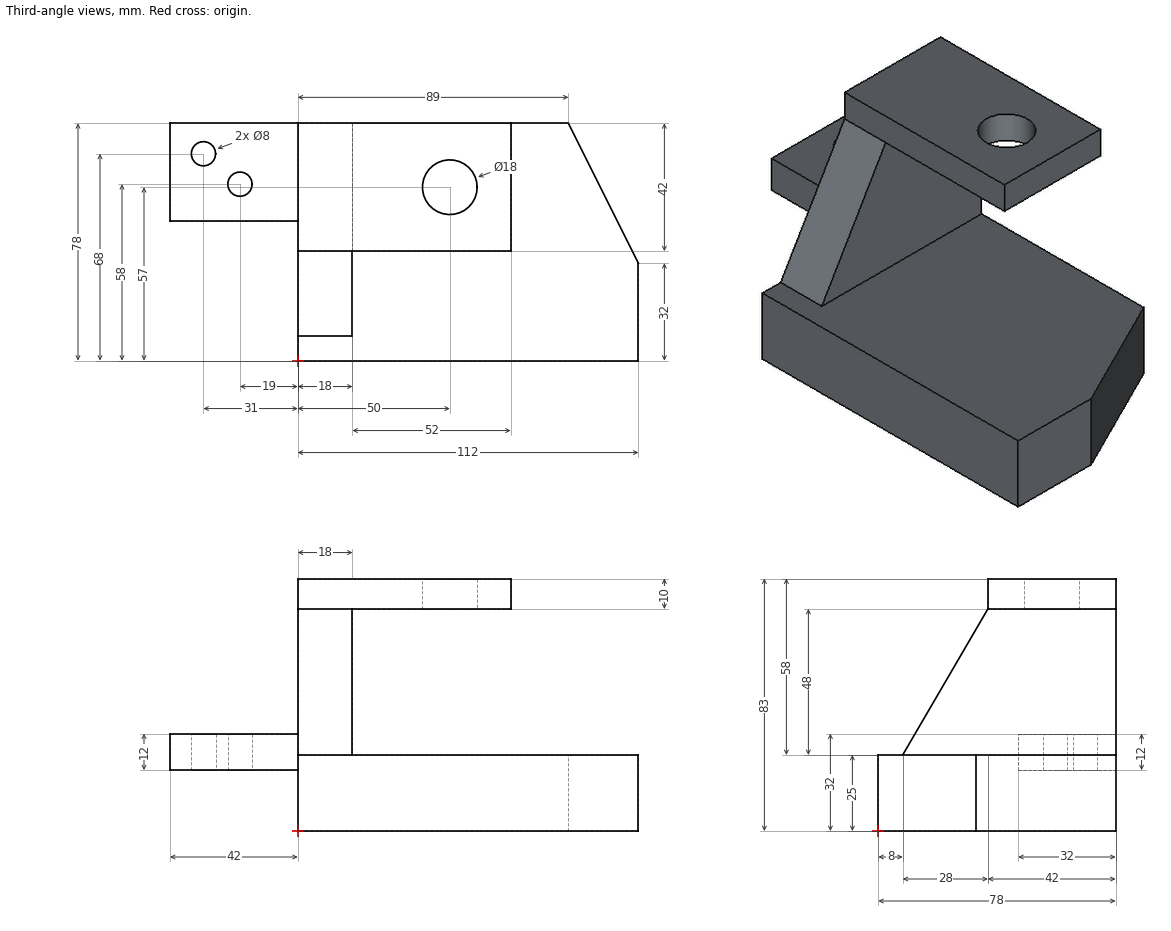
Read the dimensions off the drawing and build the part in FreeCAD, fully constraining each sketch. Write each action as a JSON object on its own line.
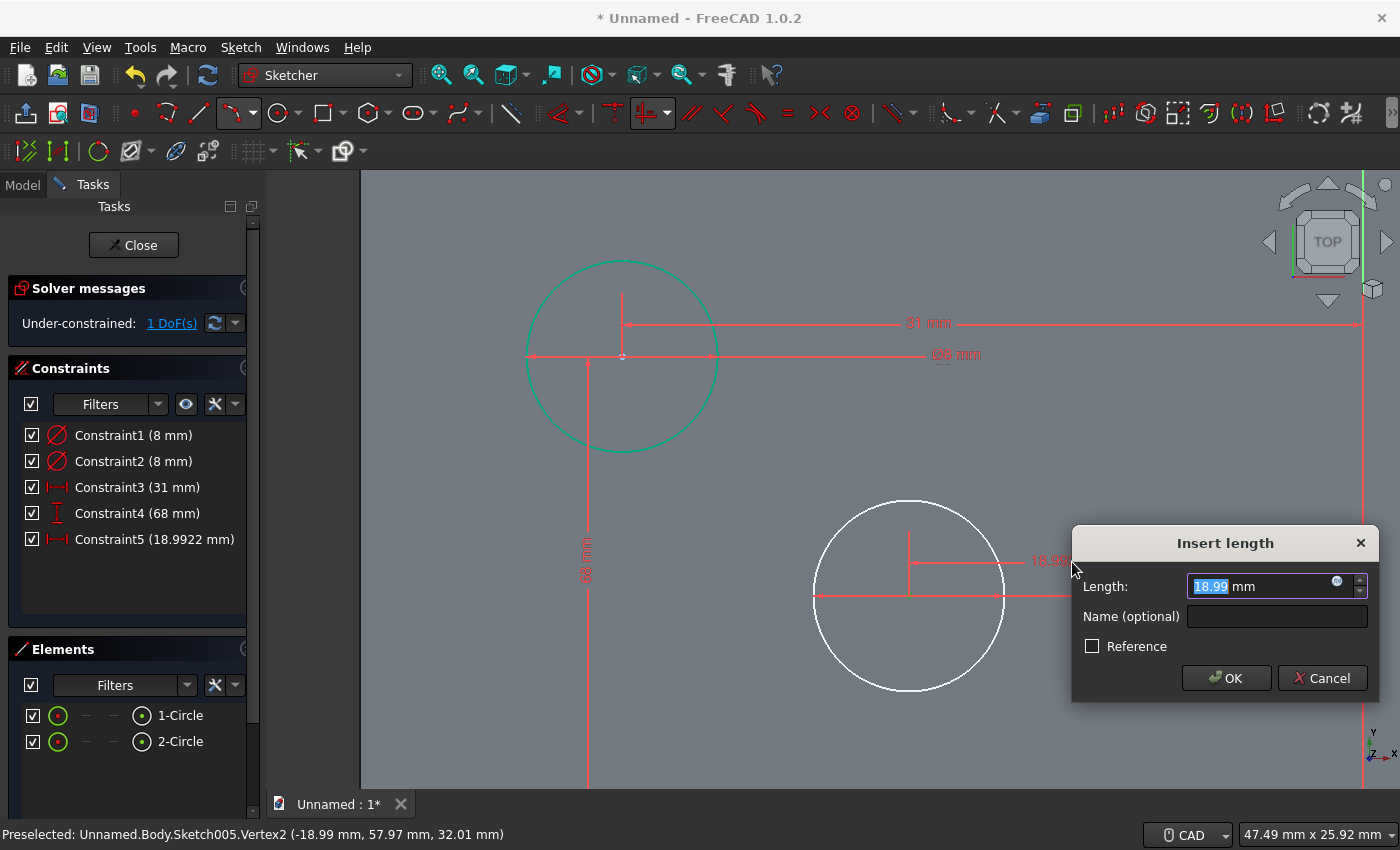
{"action": "type", "text": "19"}
{"action": "key", "text": "Return"}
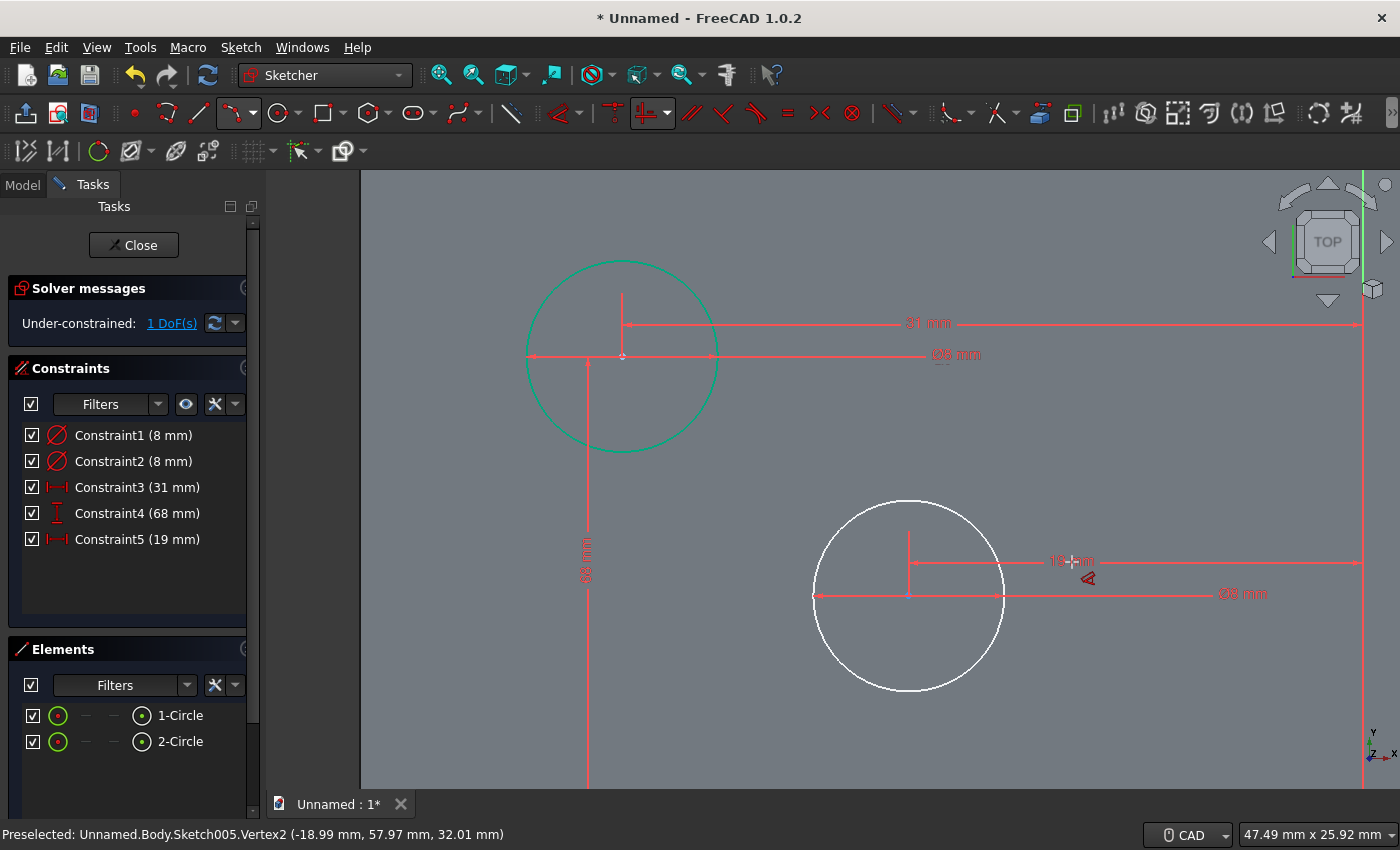
{"action": "left_click", "coordinate": [909, 596]}
{"action": "left_click", "coordinate": [875, 641]}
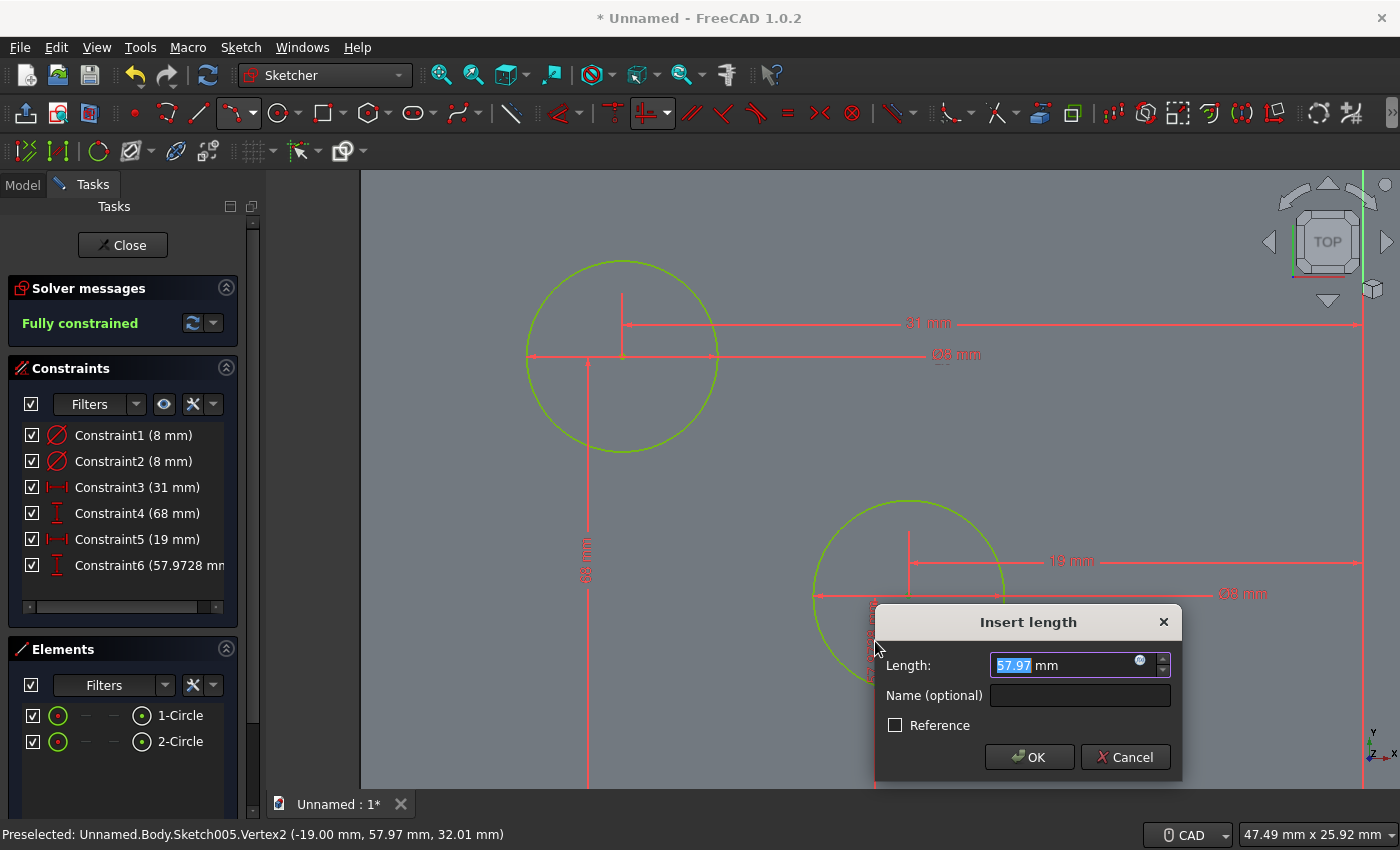
{"action": "type", "text": "58"}
{"action": "key", "text": "Return"}
{"action": "key", "text": "Escape"}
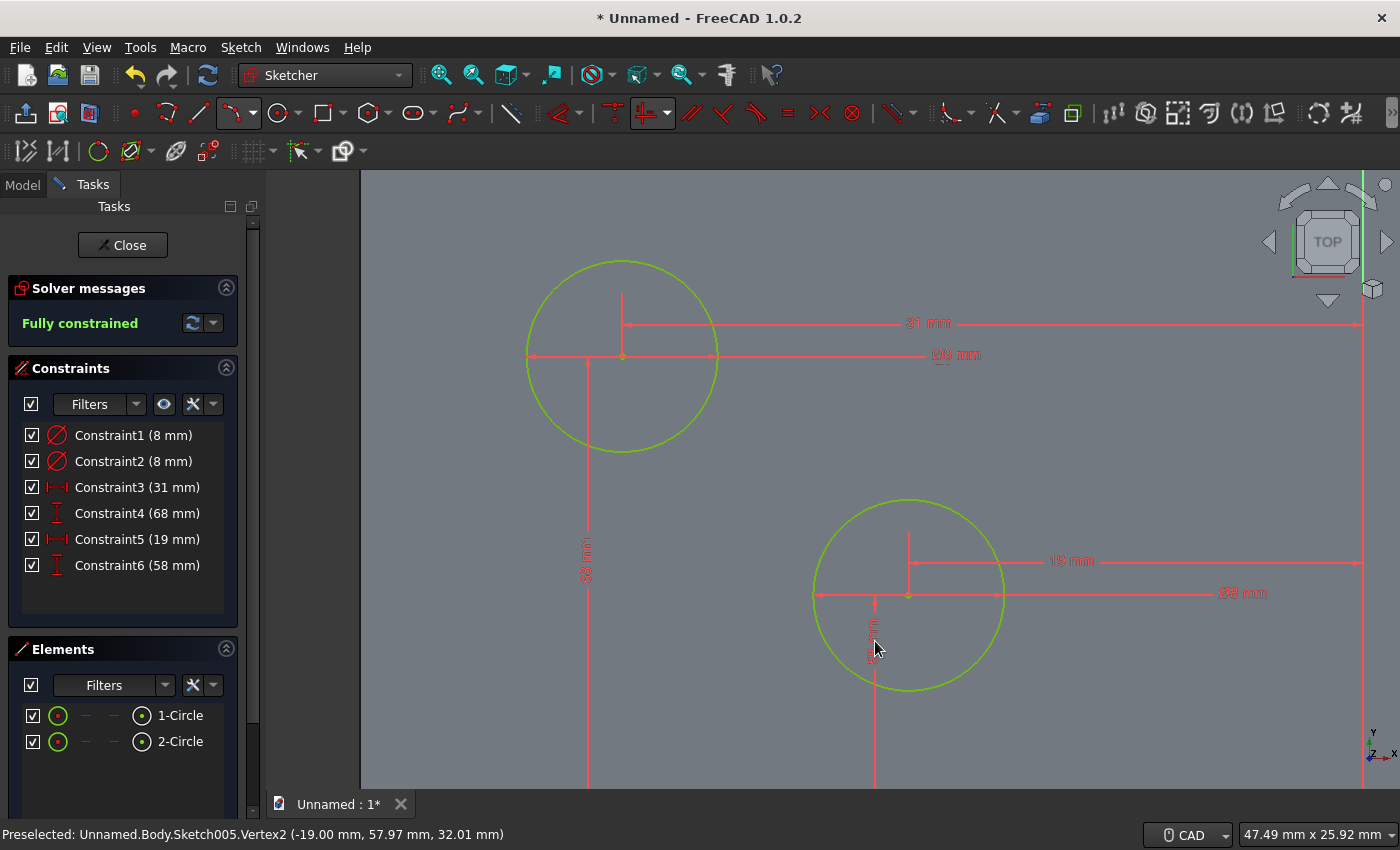
{"action": "left_click", "coordinate": [123, 245]}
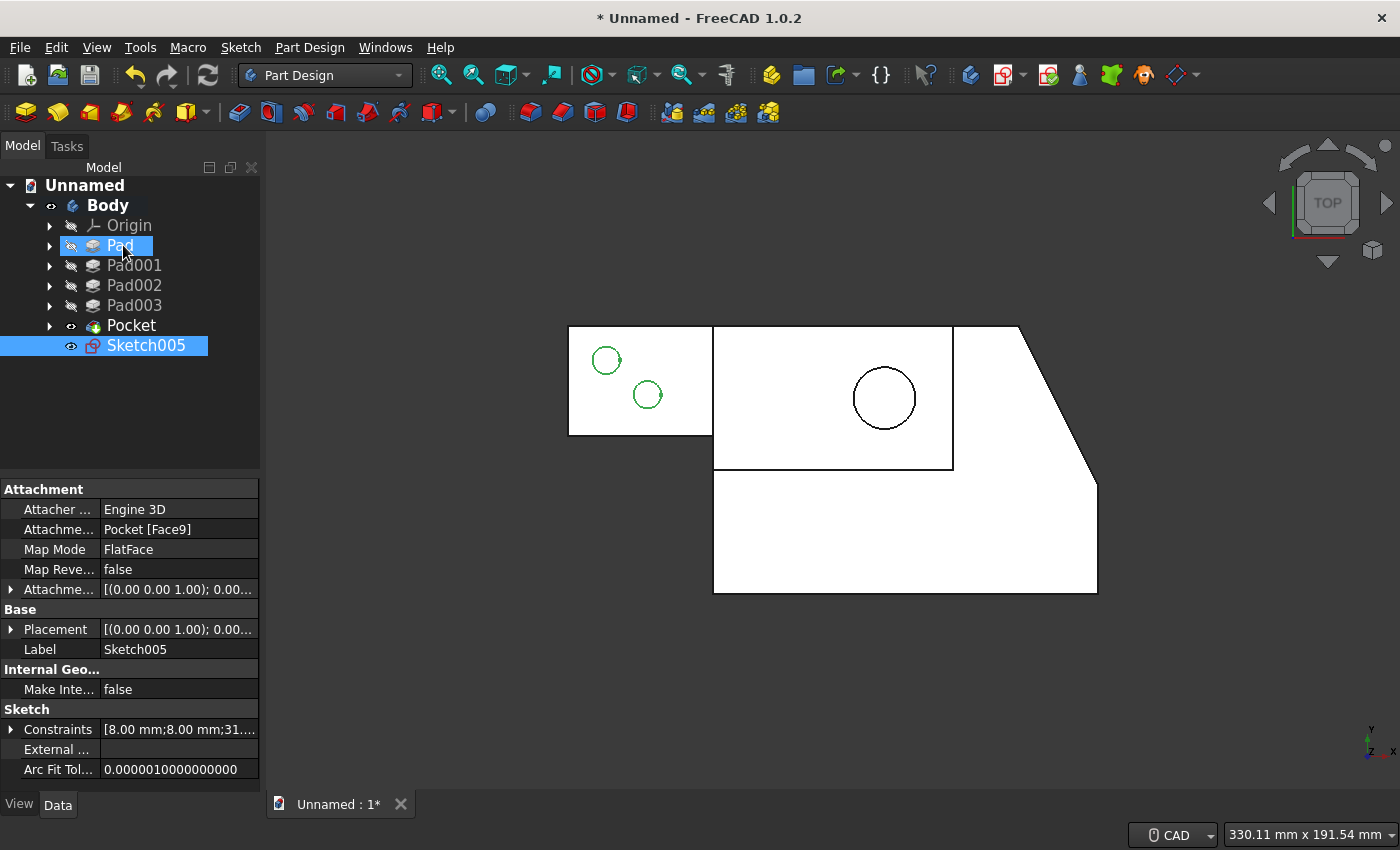
{"action": "left_click", "coordinate": [240, 112]}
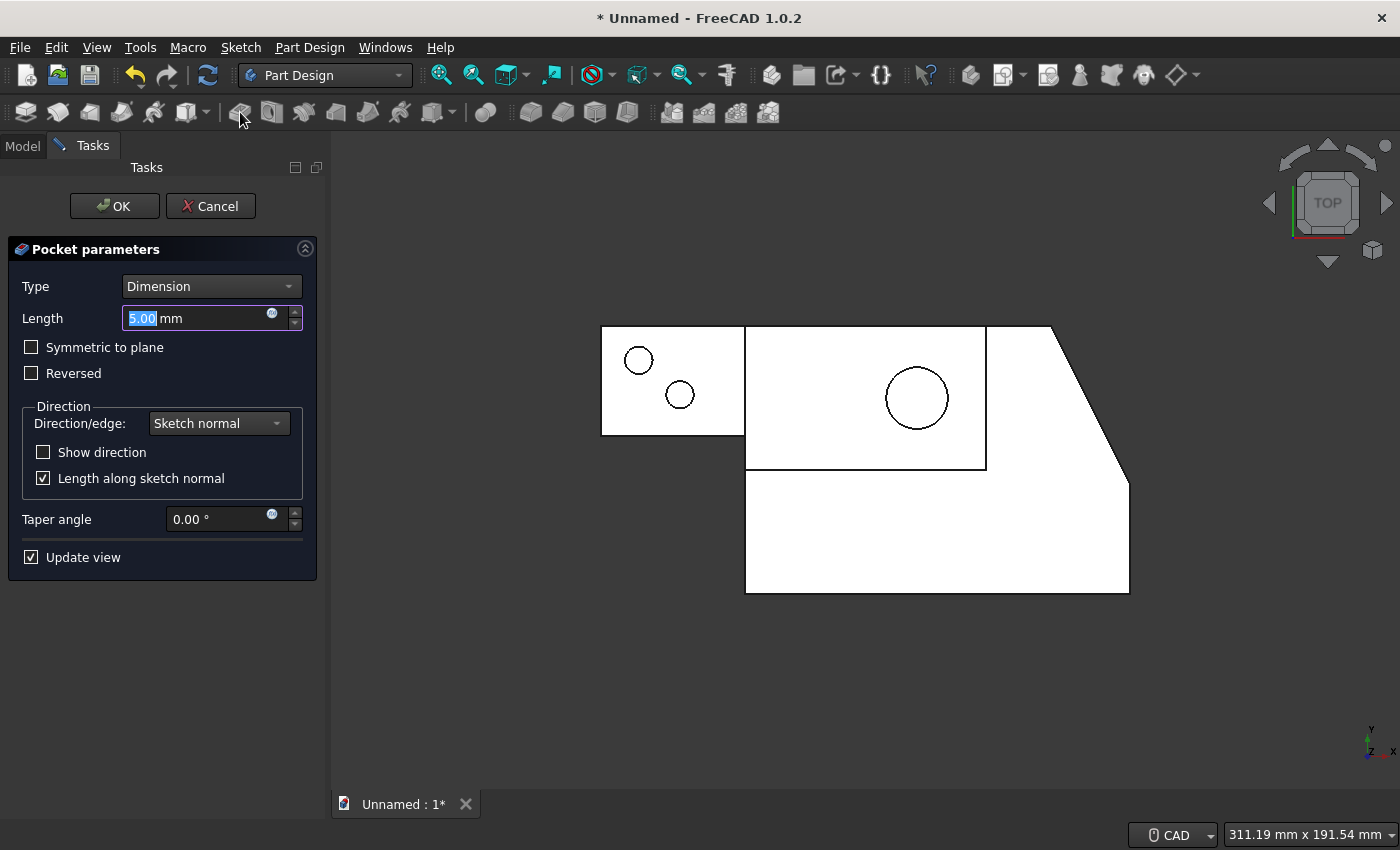
{"action": "type", "text": "12"}
{"action": "key", "text": "Tab"}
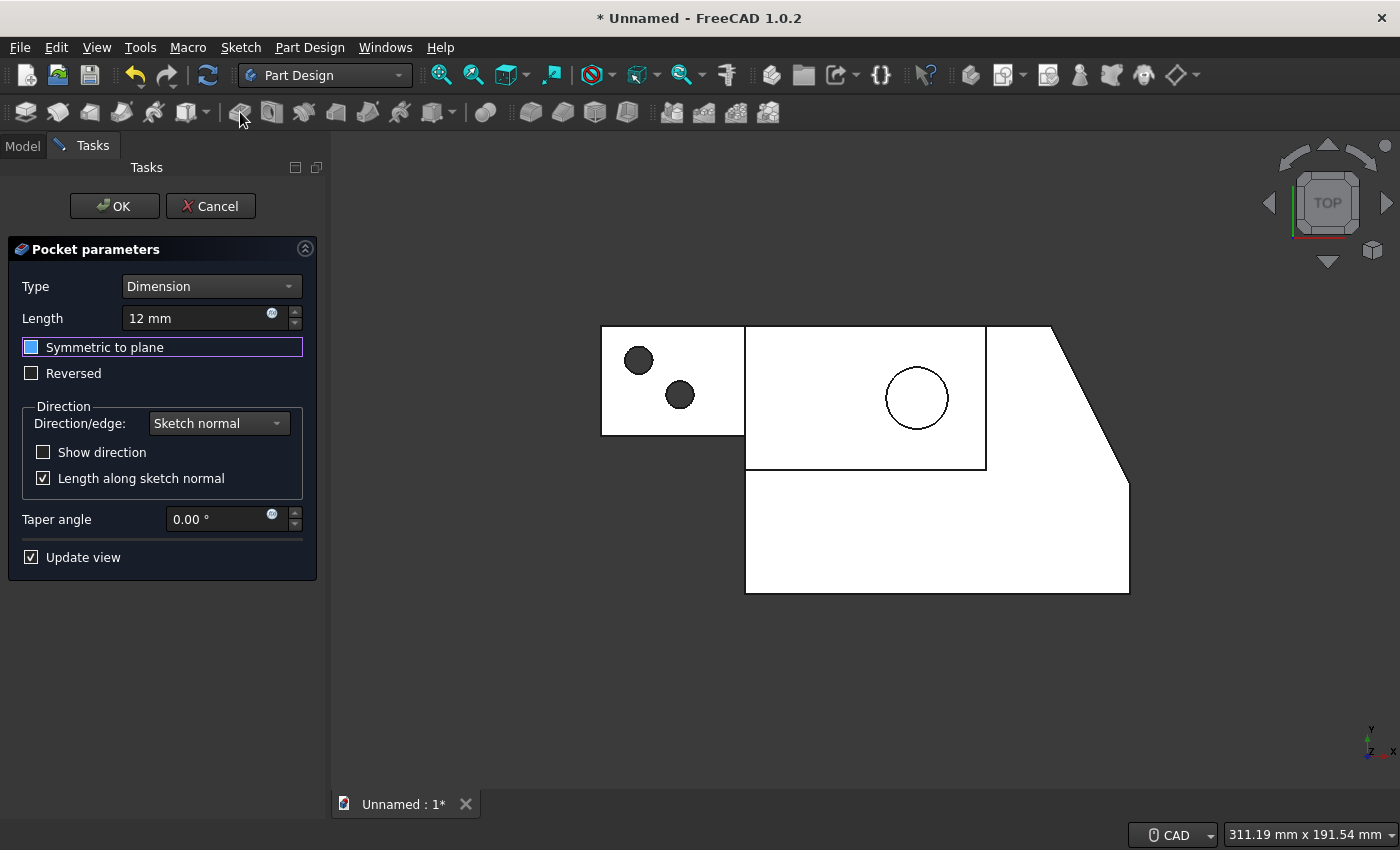
{"action": "left_click", "coordinate": [115, 206]}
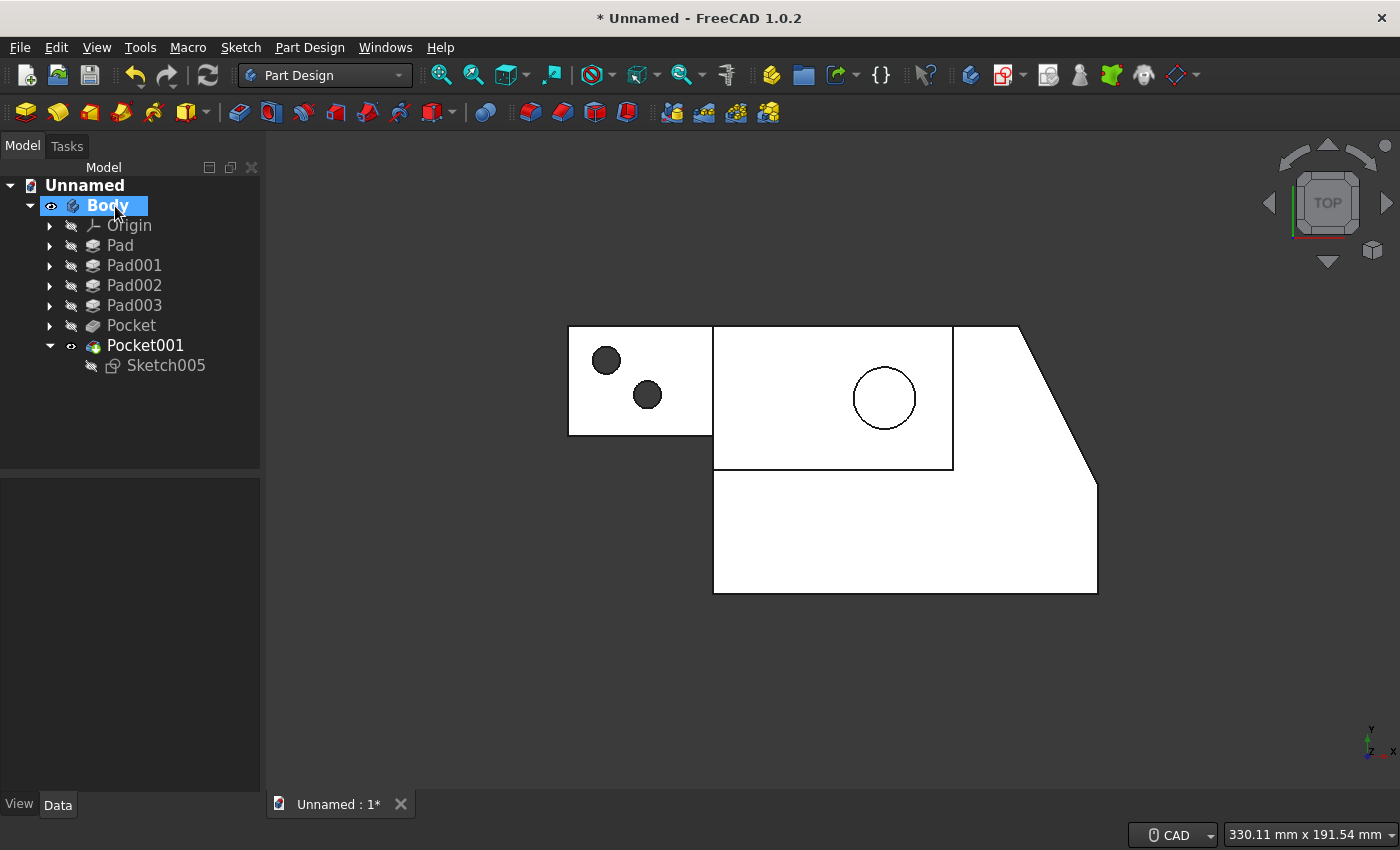
{"action": "key", "text": "6"}